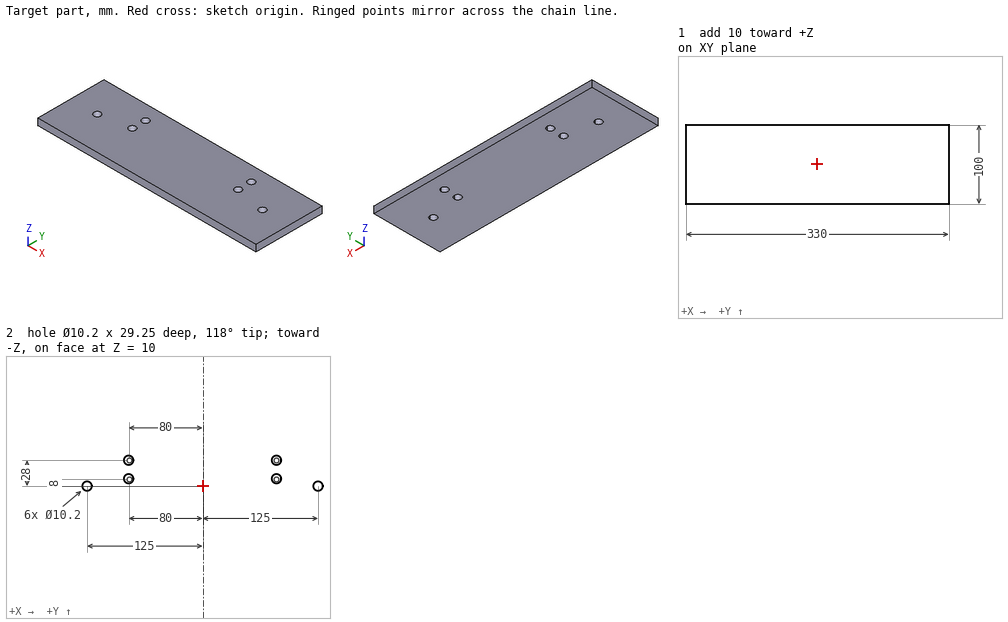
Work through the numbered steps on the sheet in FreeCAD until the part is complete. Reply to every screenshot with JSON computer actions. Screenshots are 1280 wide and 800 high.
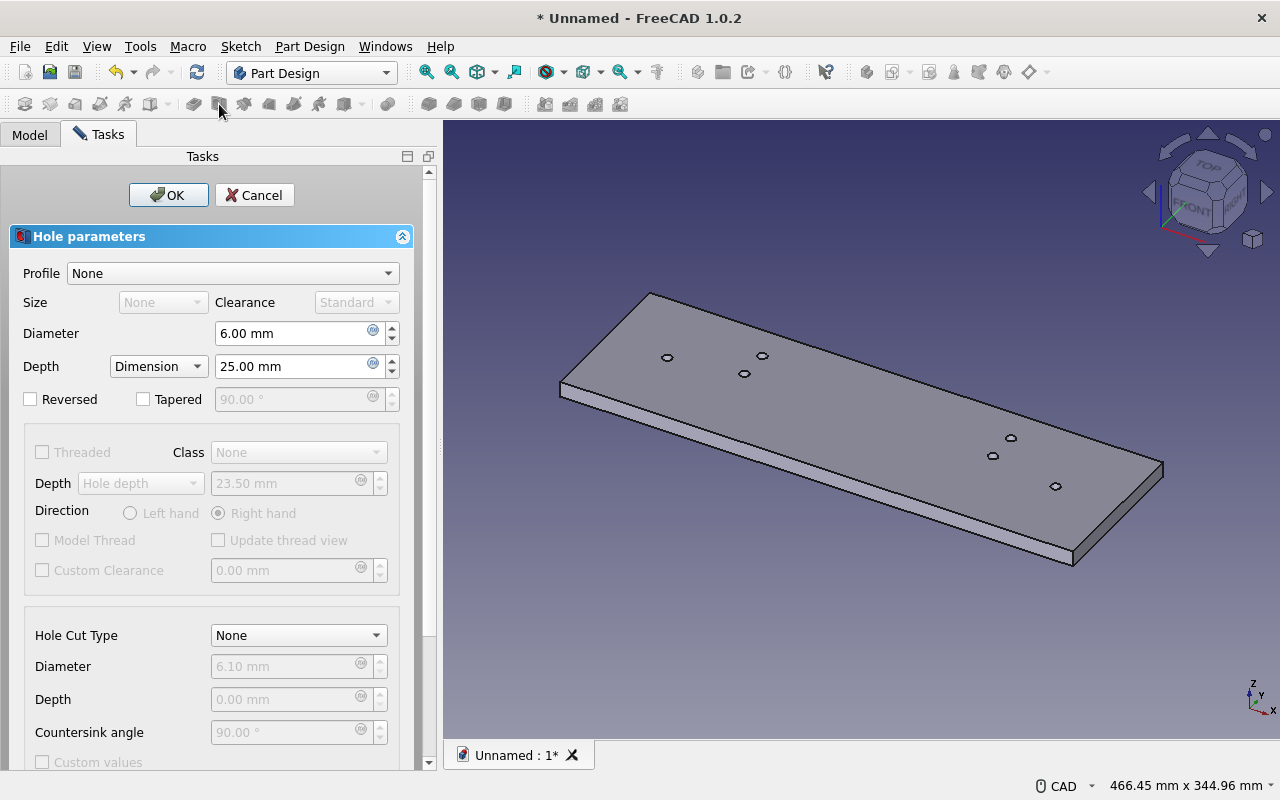
{"action": "triple_click", "coordinate": [300, 334]}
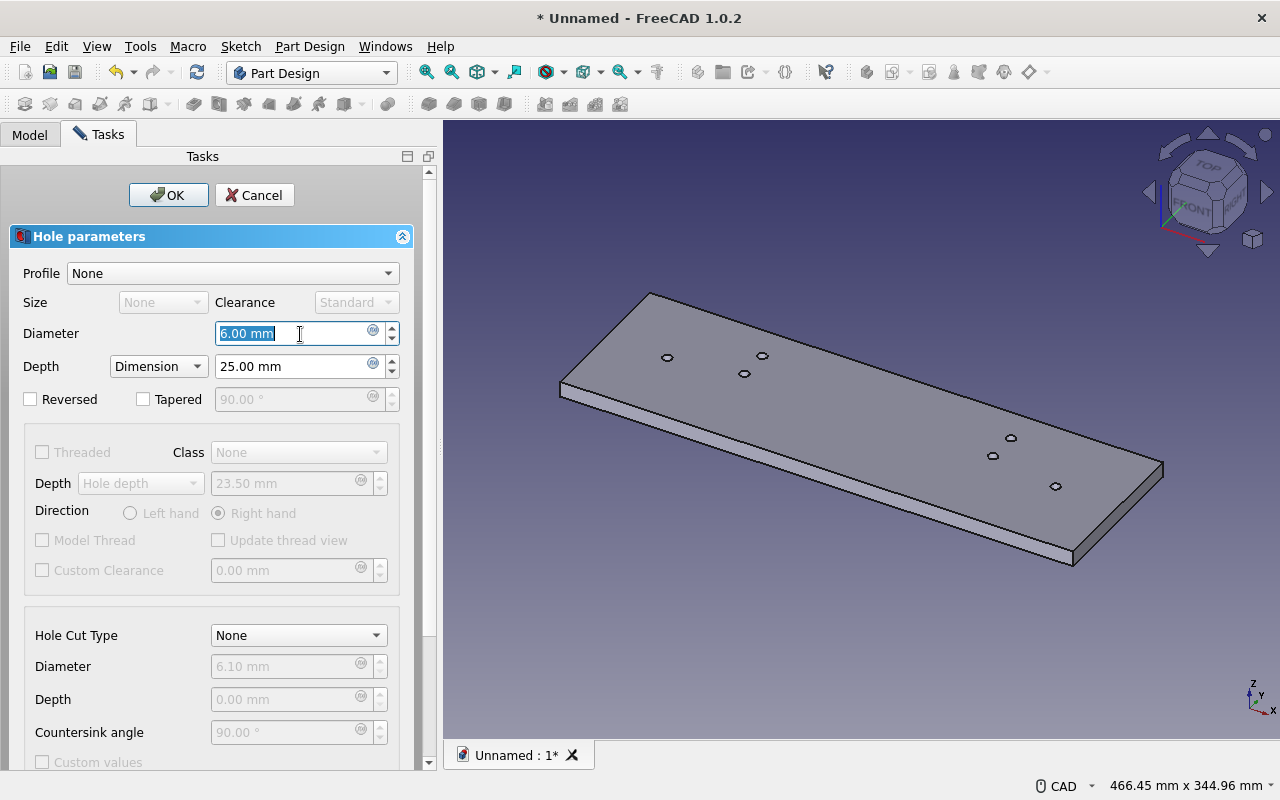
{"action": "type", "text": "10.2"}
{"action": "key", "text": "Tab"}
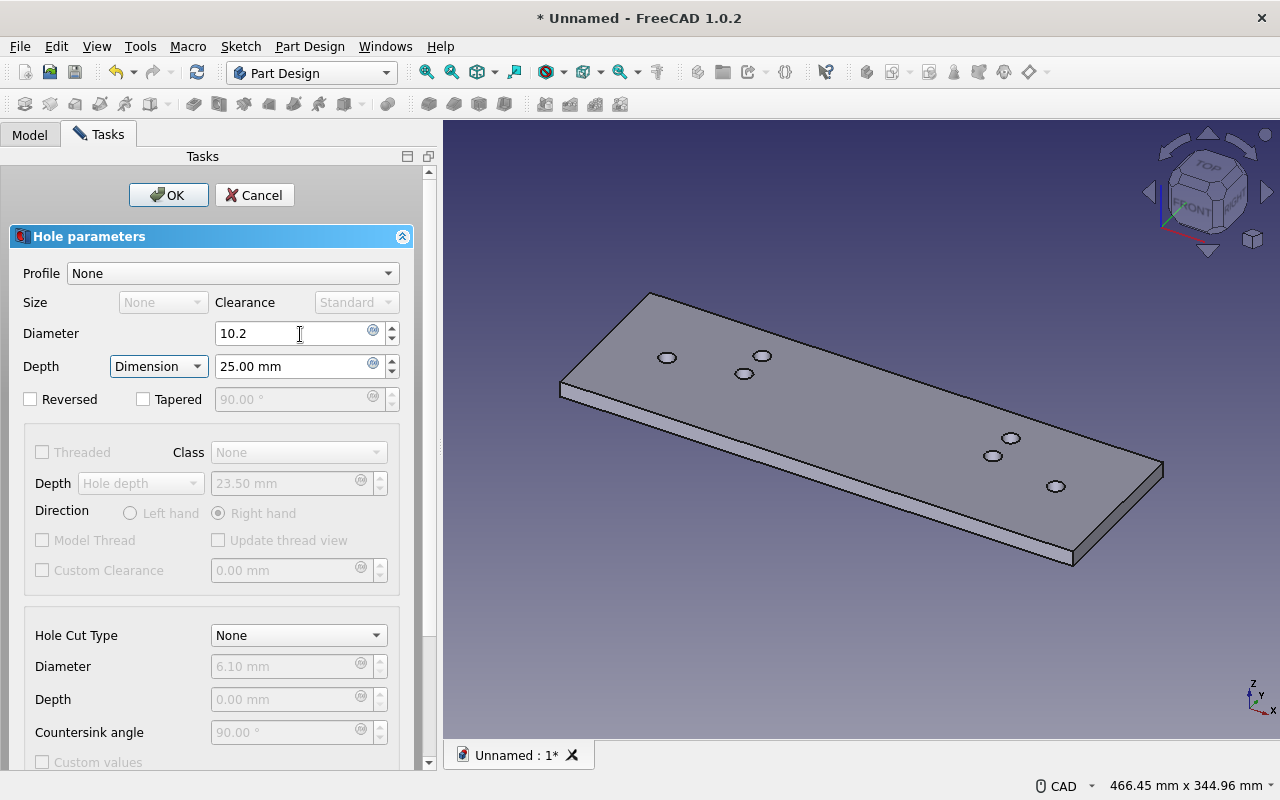
{"action": "triple_click", "coordinate": [300, 366]}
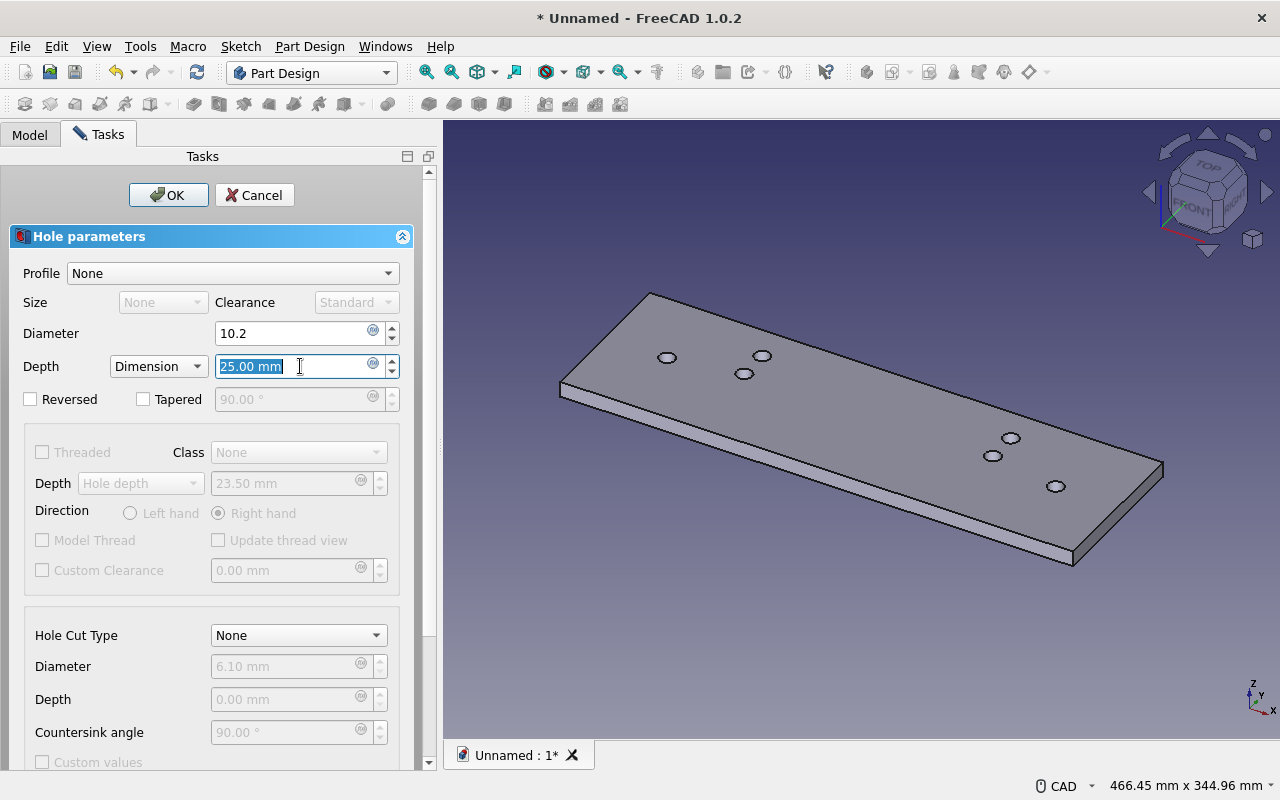
{"action": "type", "text": "29.25"}
{"action": "key", "text": "Tab"}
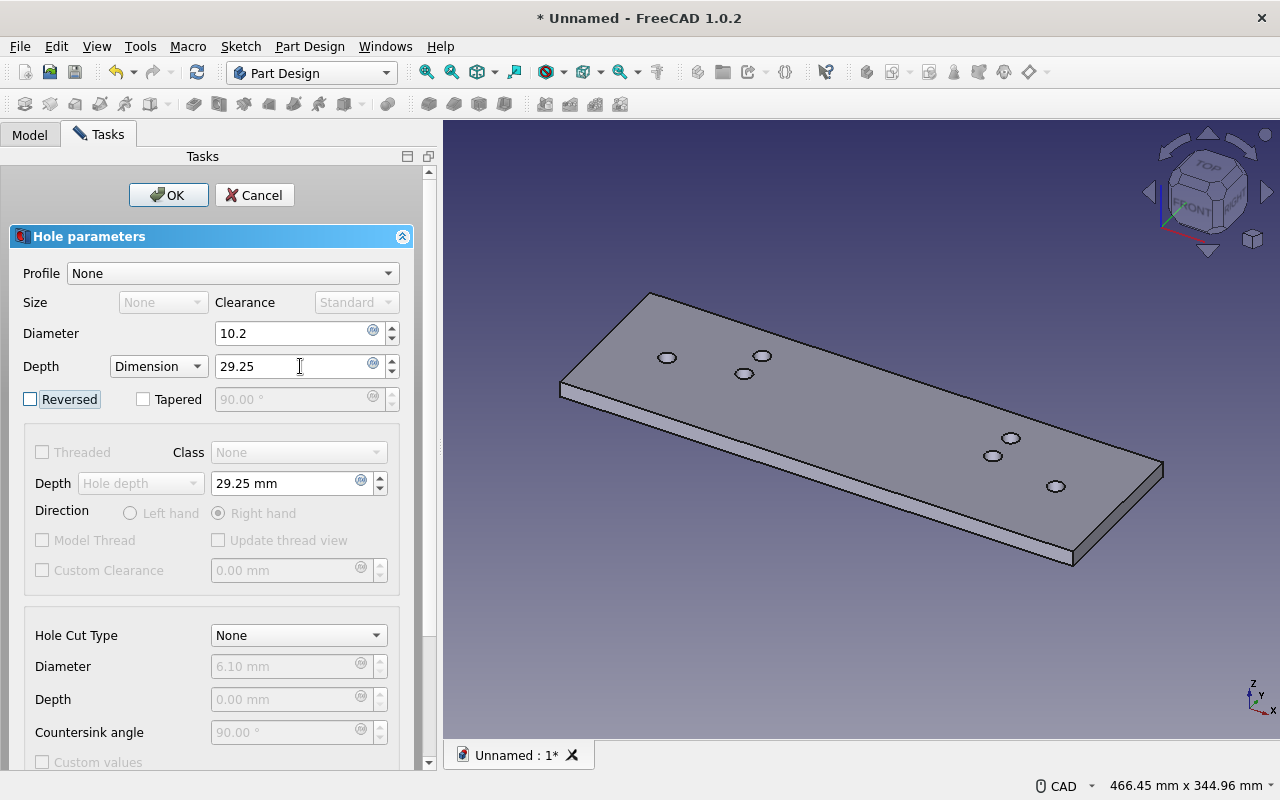
{"action": "left_click", "coordinate": [169, 195]}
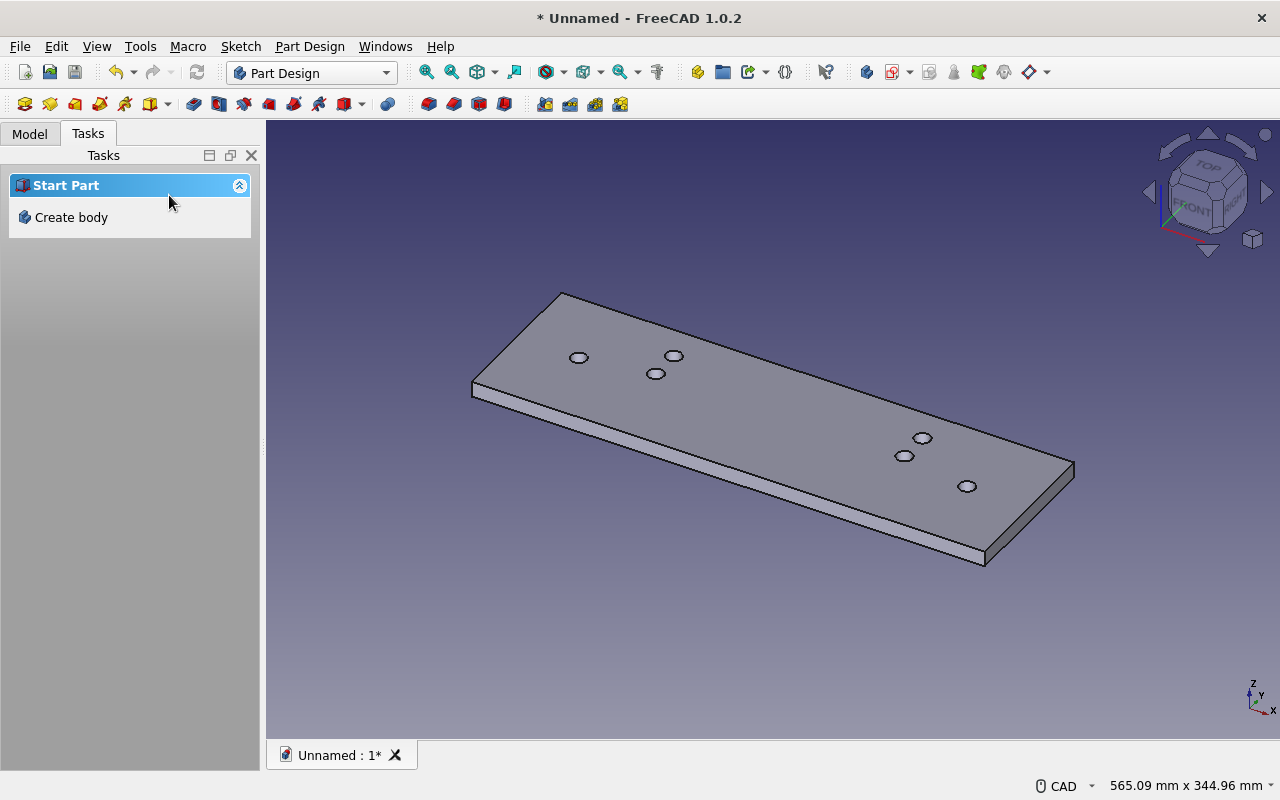
{"action": "key", "text": "0"}